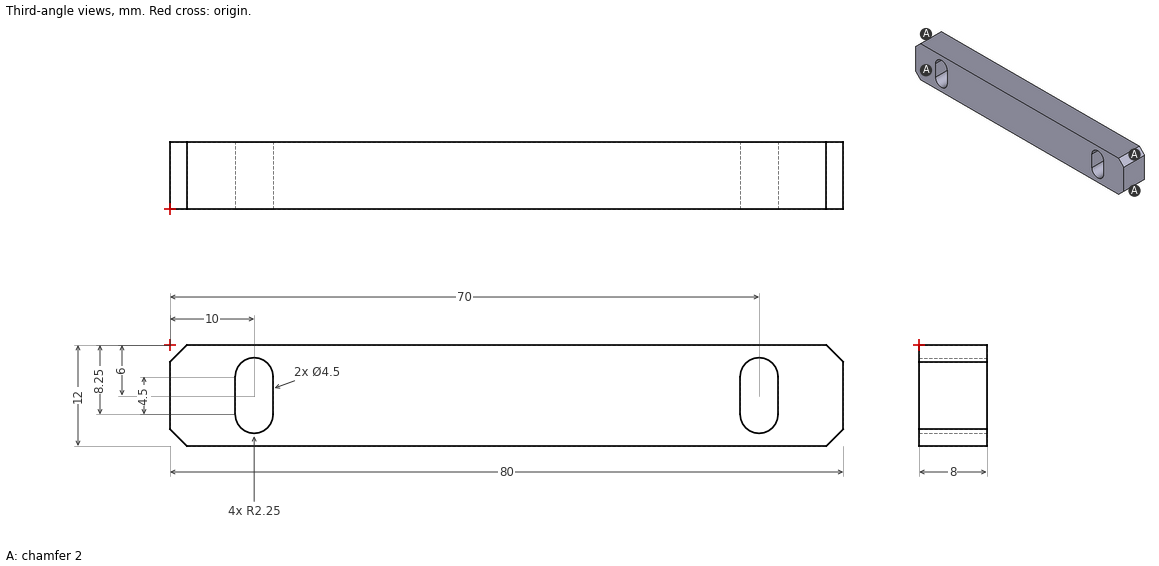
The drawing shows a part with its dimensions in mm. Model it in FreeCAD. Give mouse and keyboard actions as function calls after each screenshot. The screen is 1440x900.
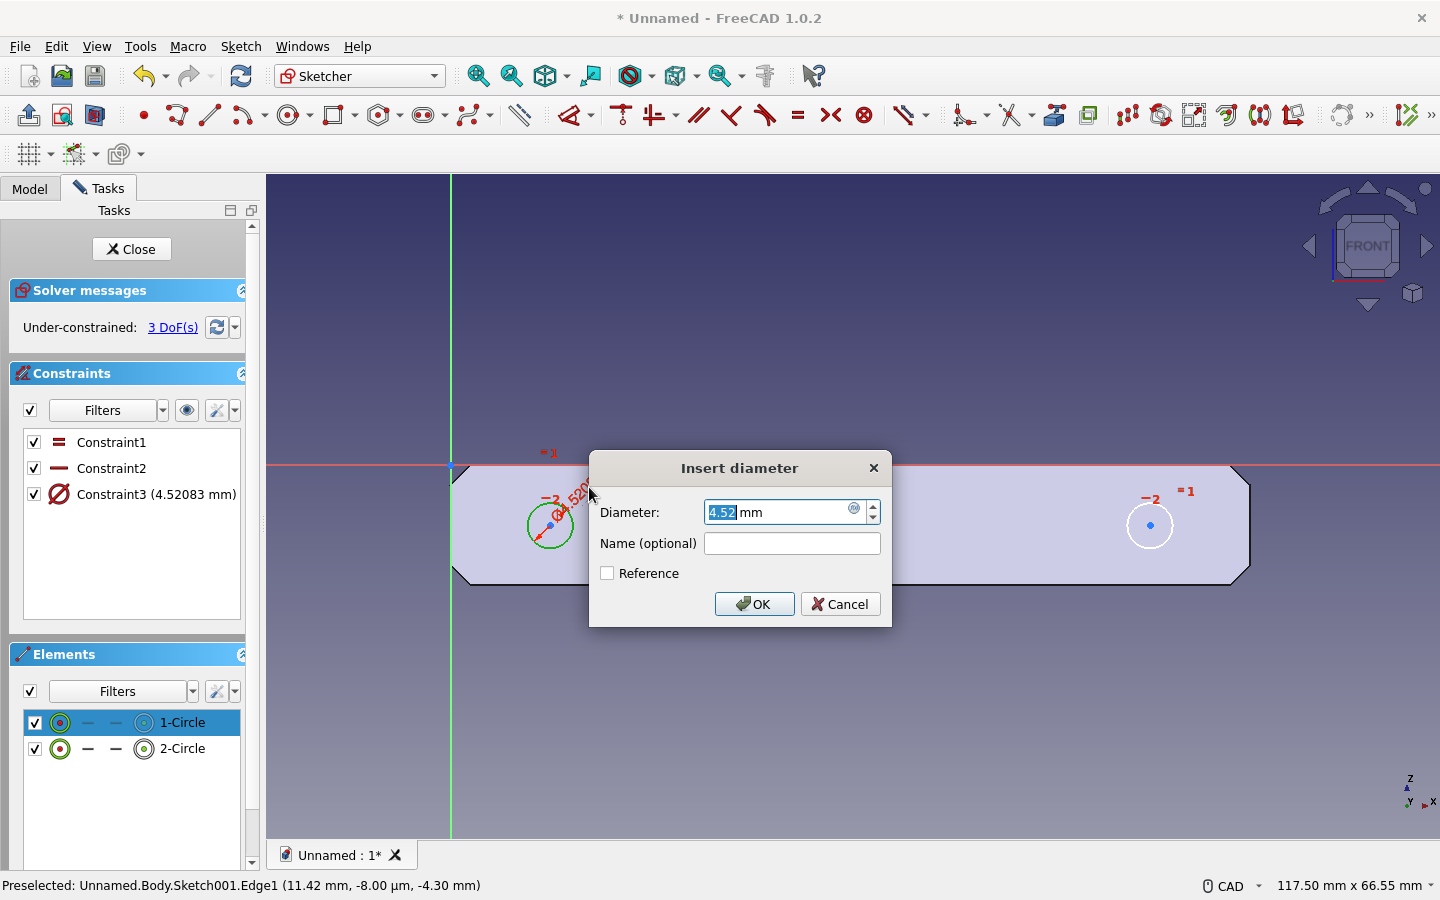
text(4.5)
key(Return)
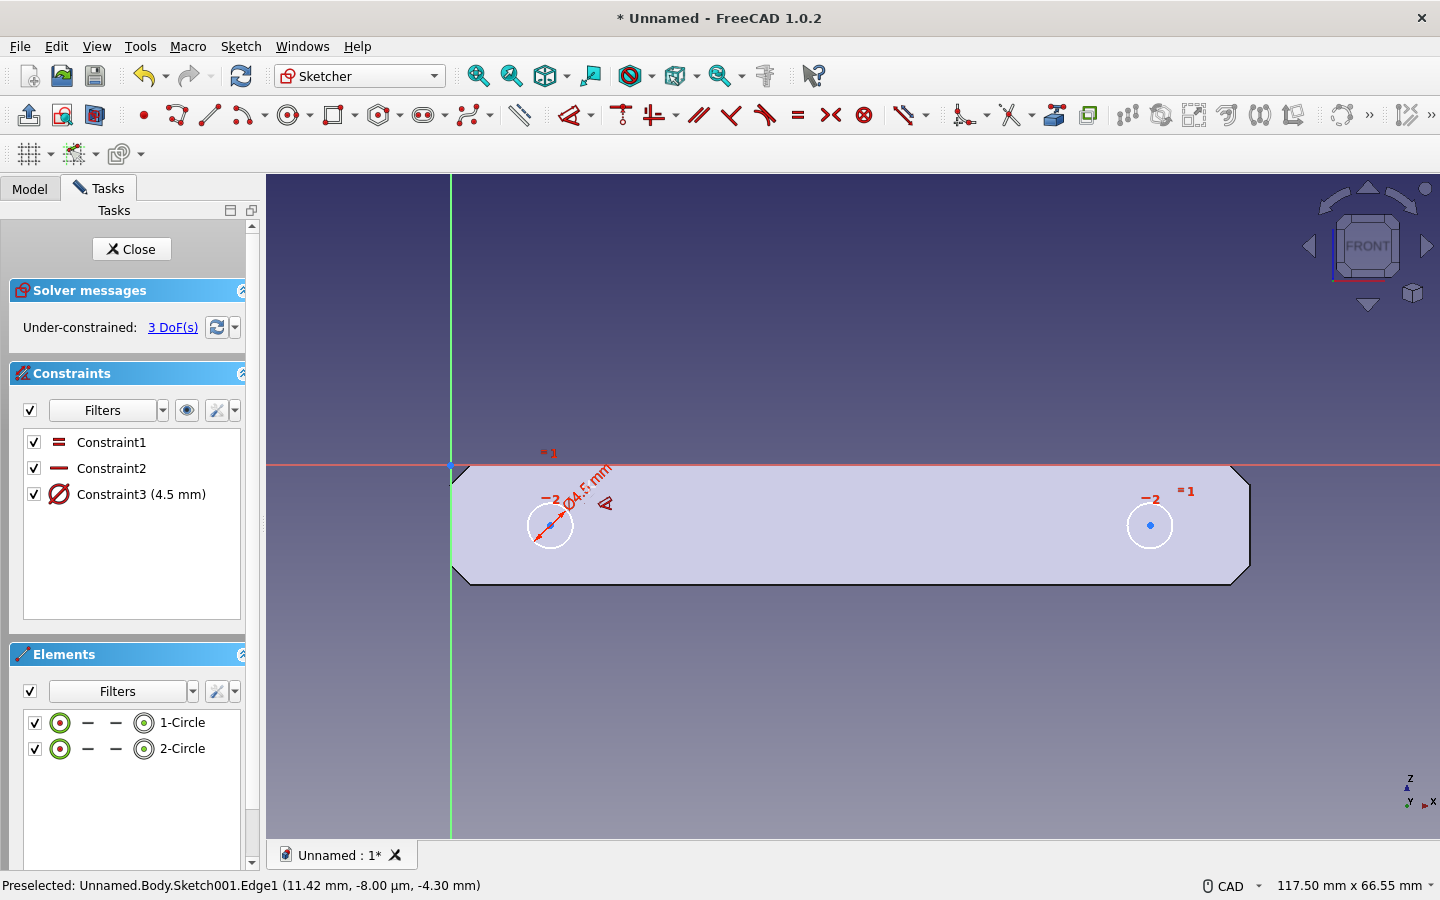
click(550, 526)
click(417, 496)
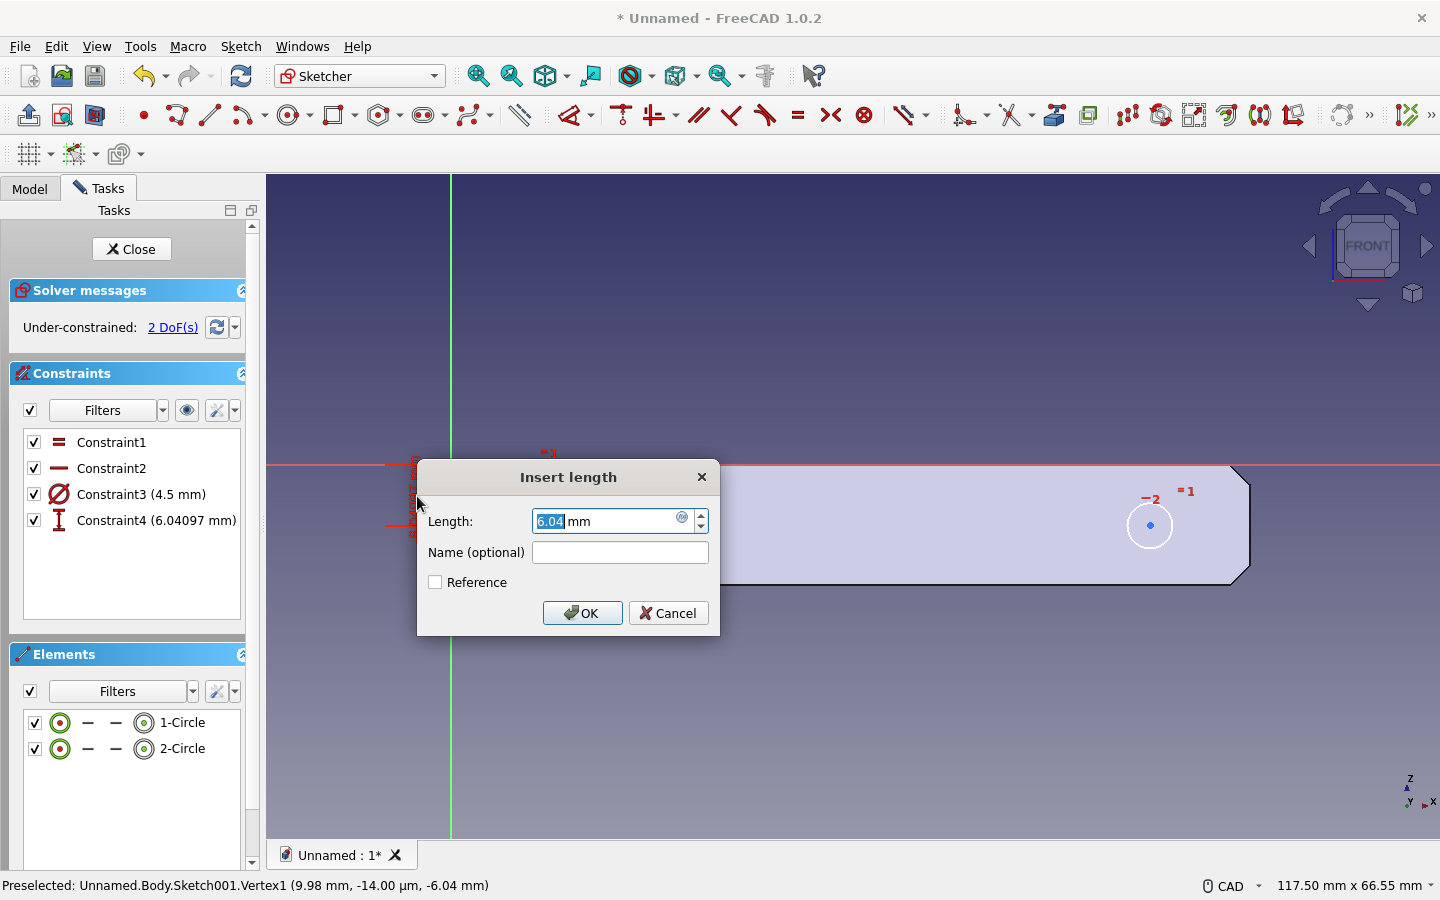
text(6)
key(Return)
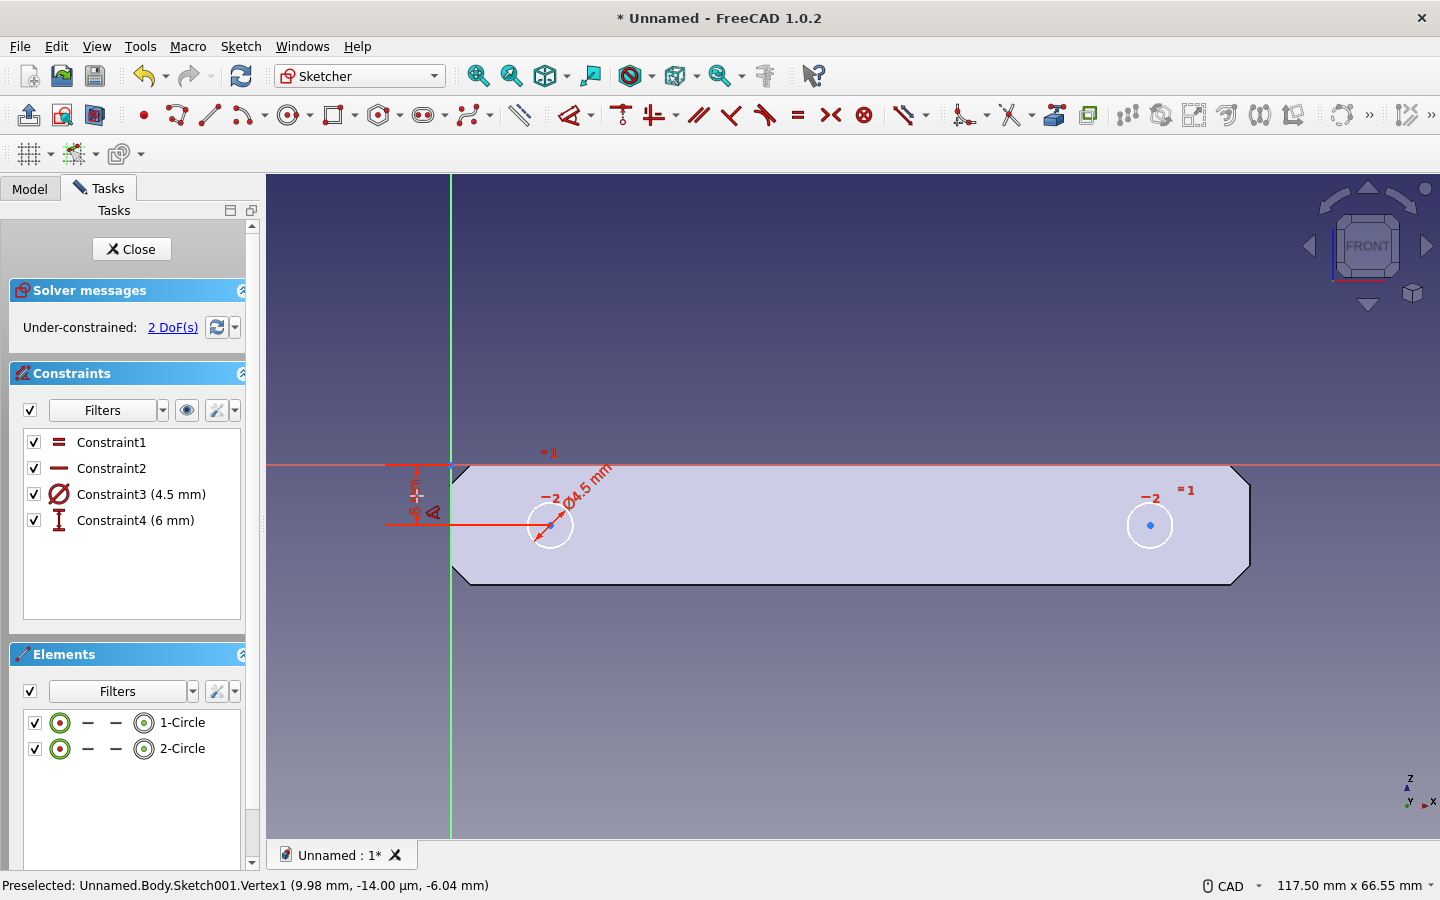
click(550, 525)
click(500, 431)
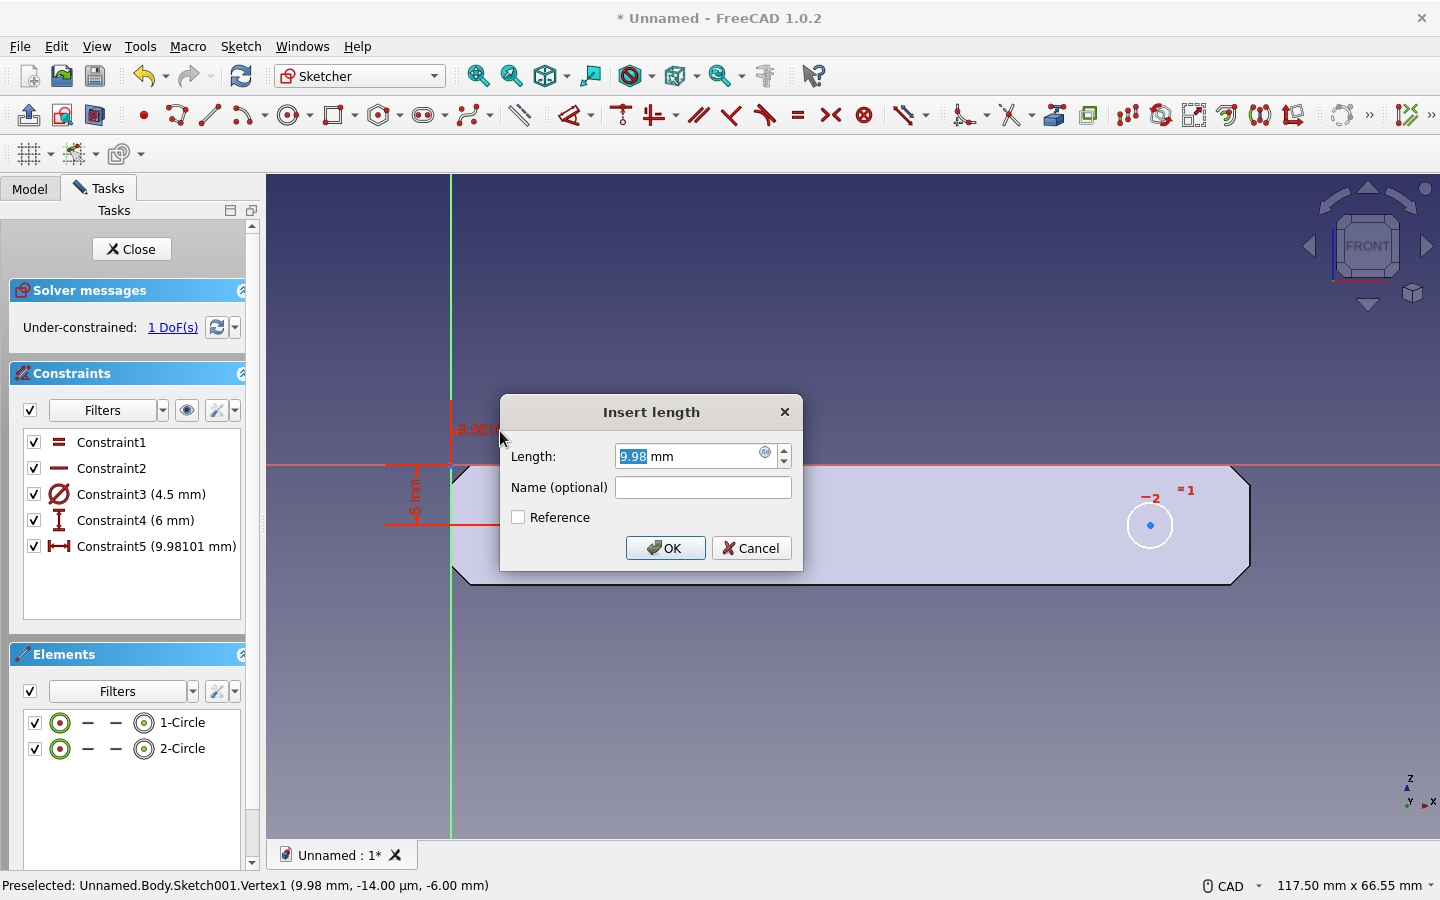
text(10)
key(Return)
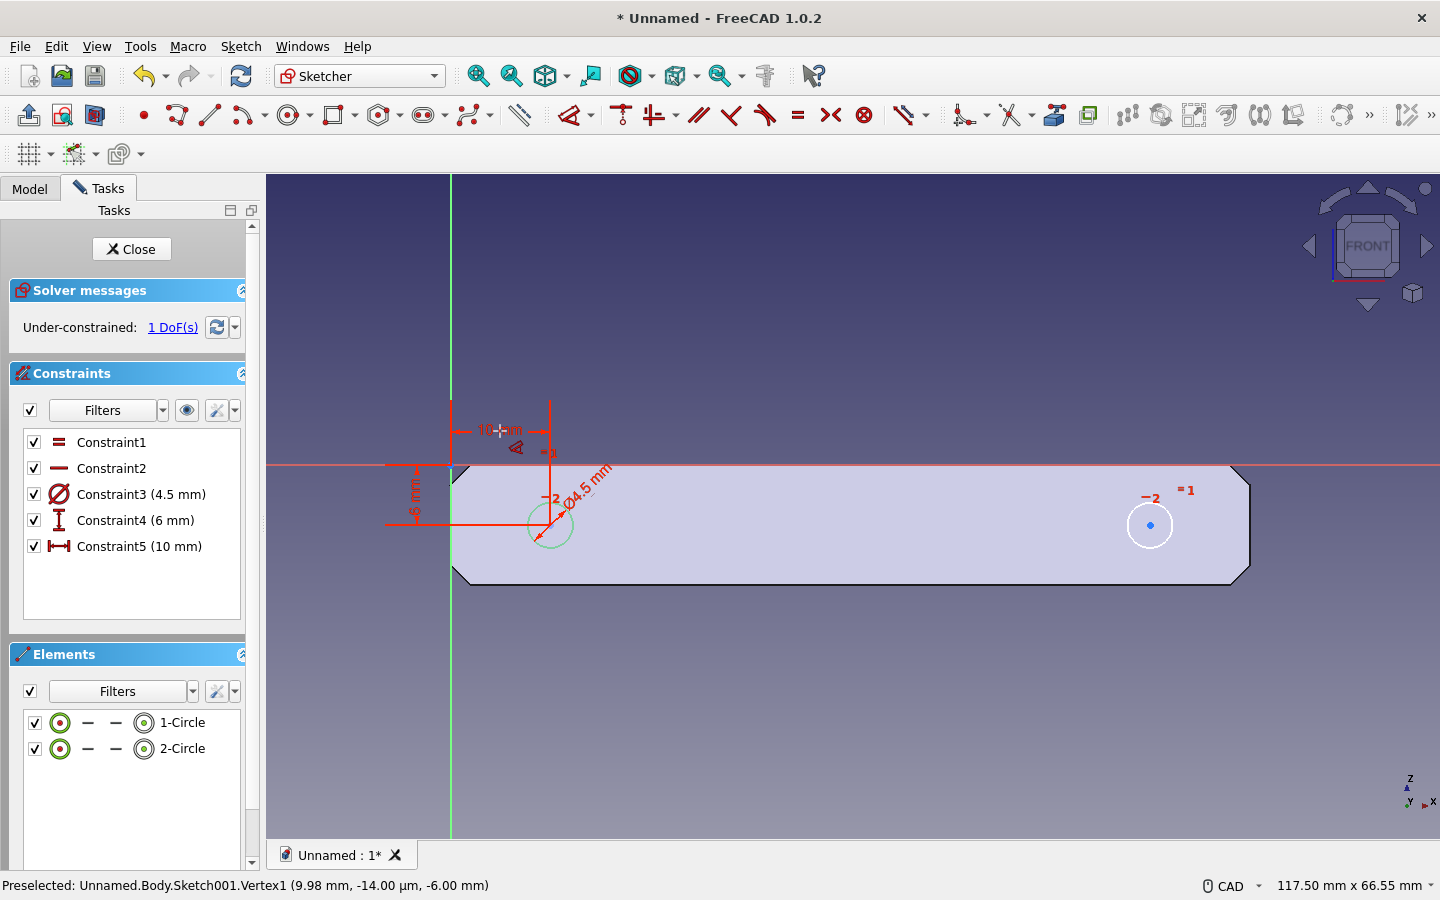
click(1150, 525)
click(800, 431)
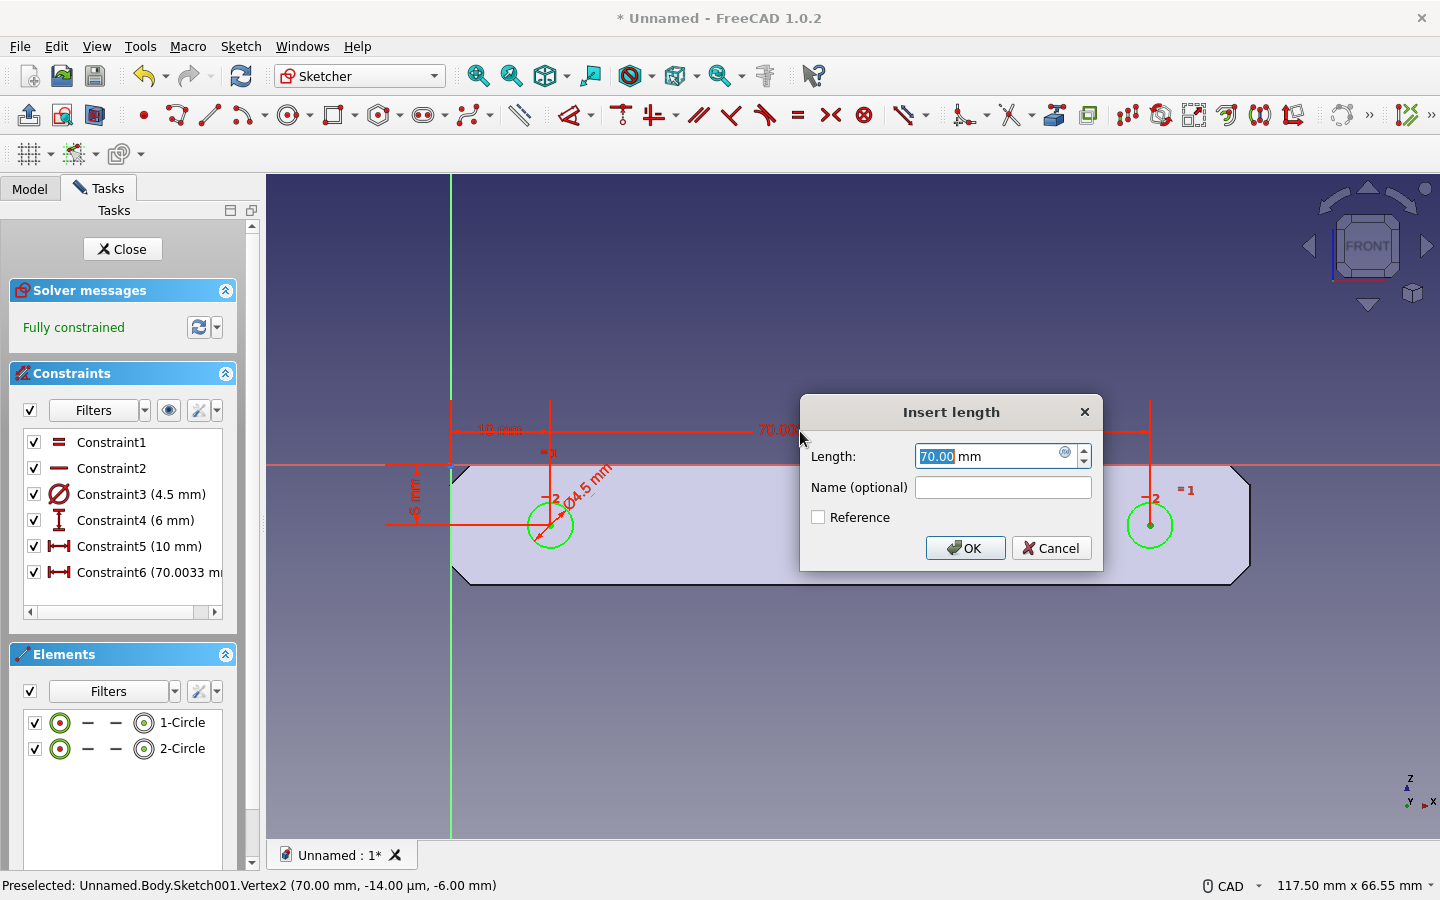
text(70)
key(Return)
key(Escape)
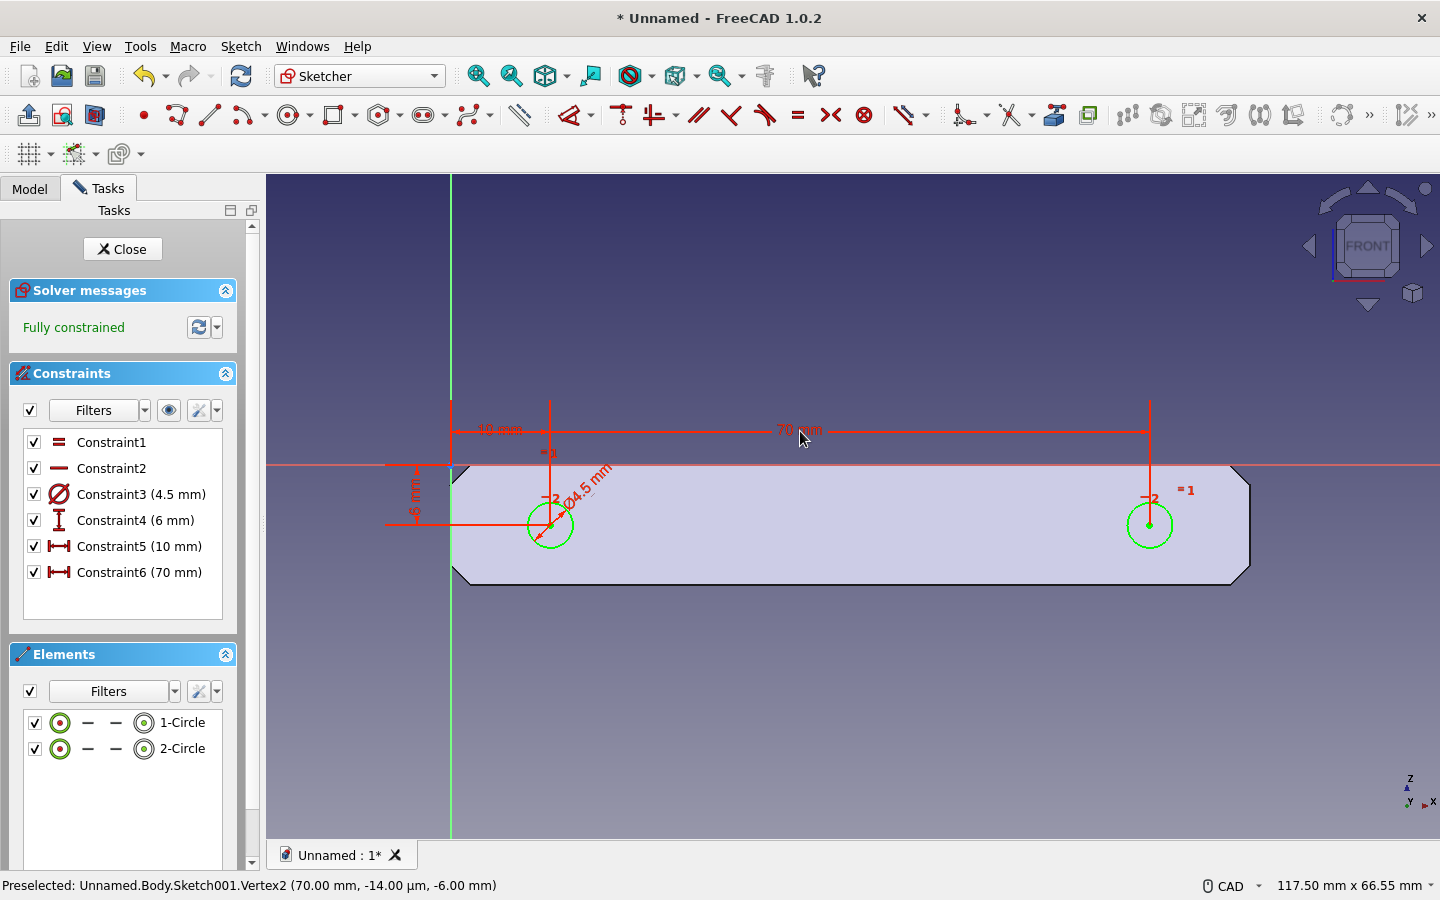
click(123, 249)